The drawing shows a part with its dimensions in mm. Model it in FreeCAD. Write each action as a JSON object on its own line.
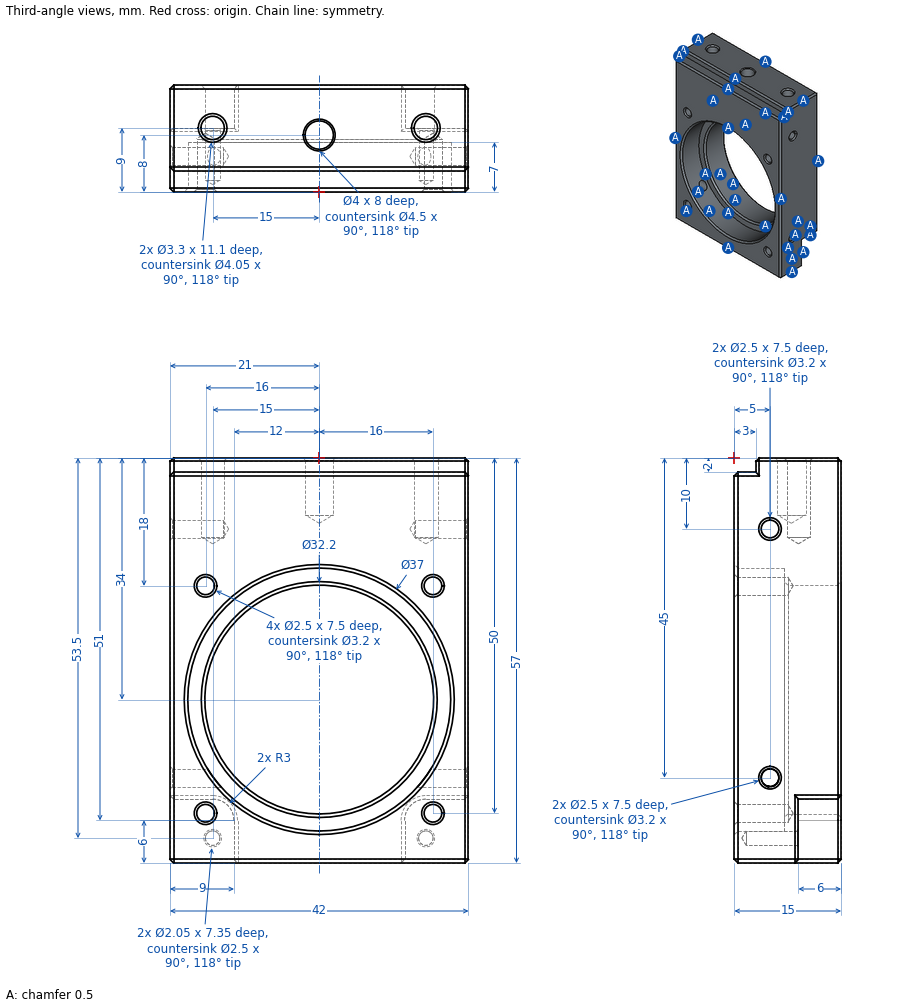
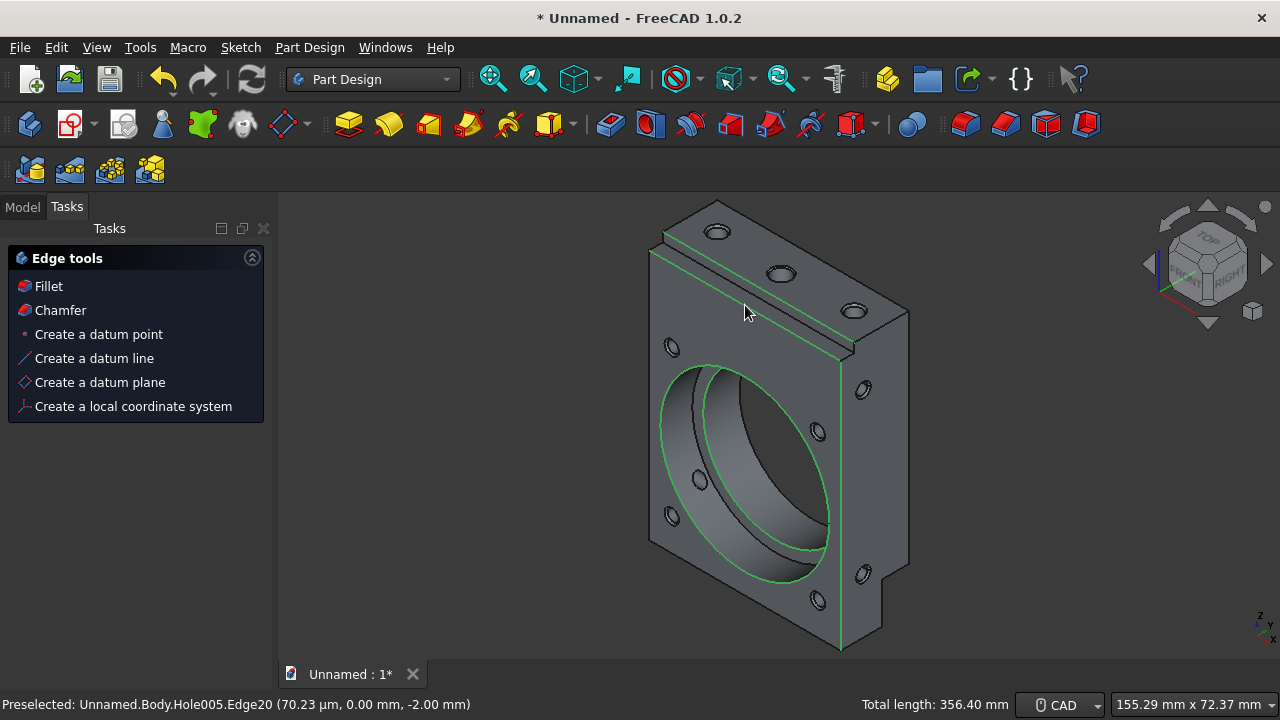
{"action": "left_click", "coordinate": [847, 356], "text": "ctrl"}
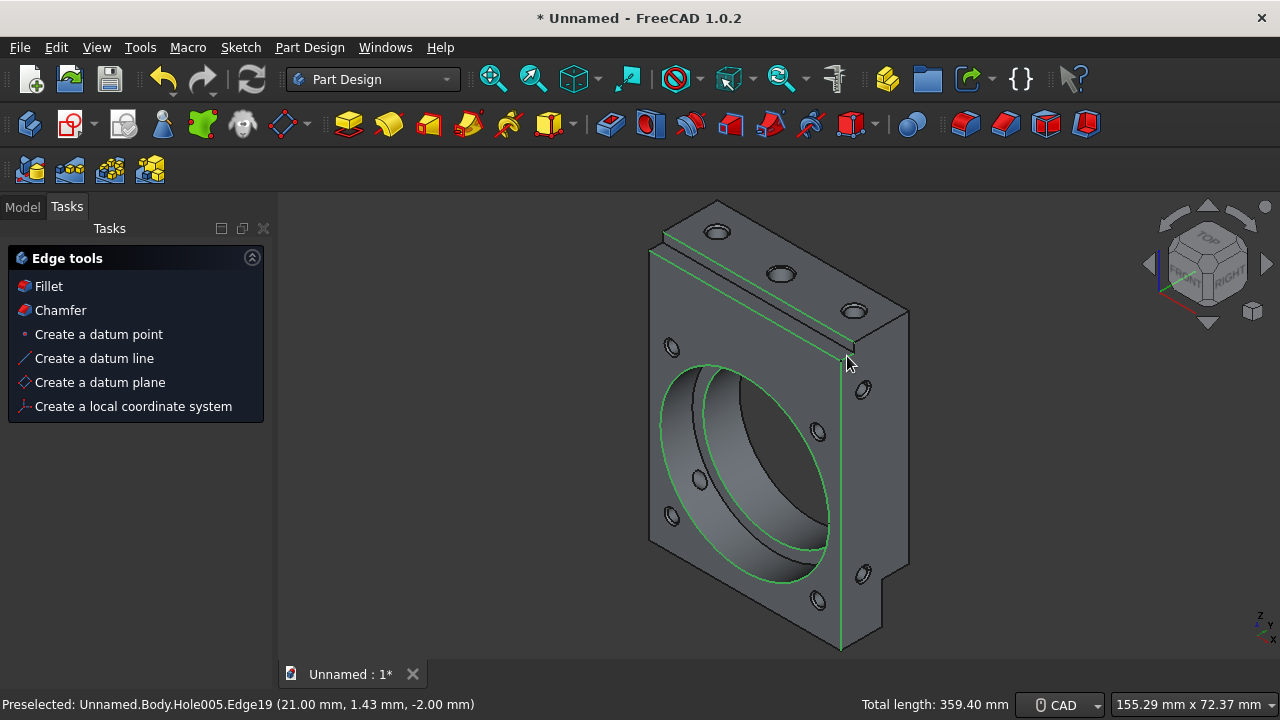
{"action": "left_click", "coordinate": [854, 348], "text": "ctrl"}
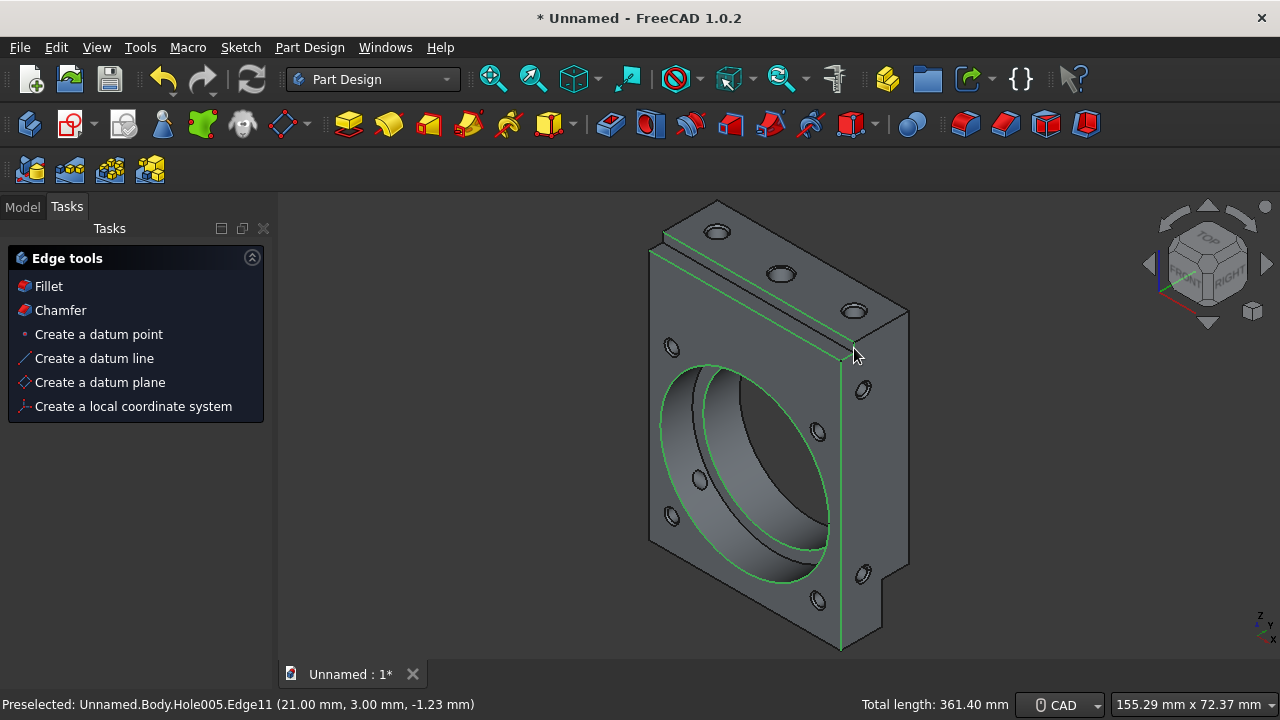
{"action": "left_click", "coordinate": [882, 326], "text": "ctrl"}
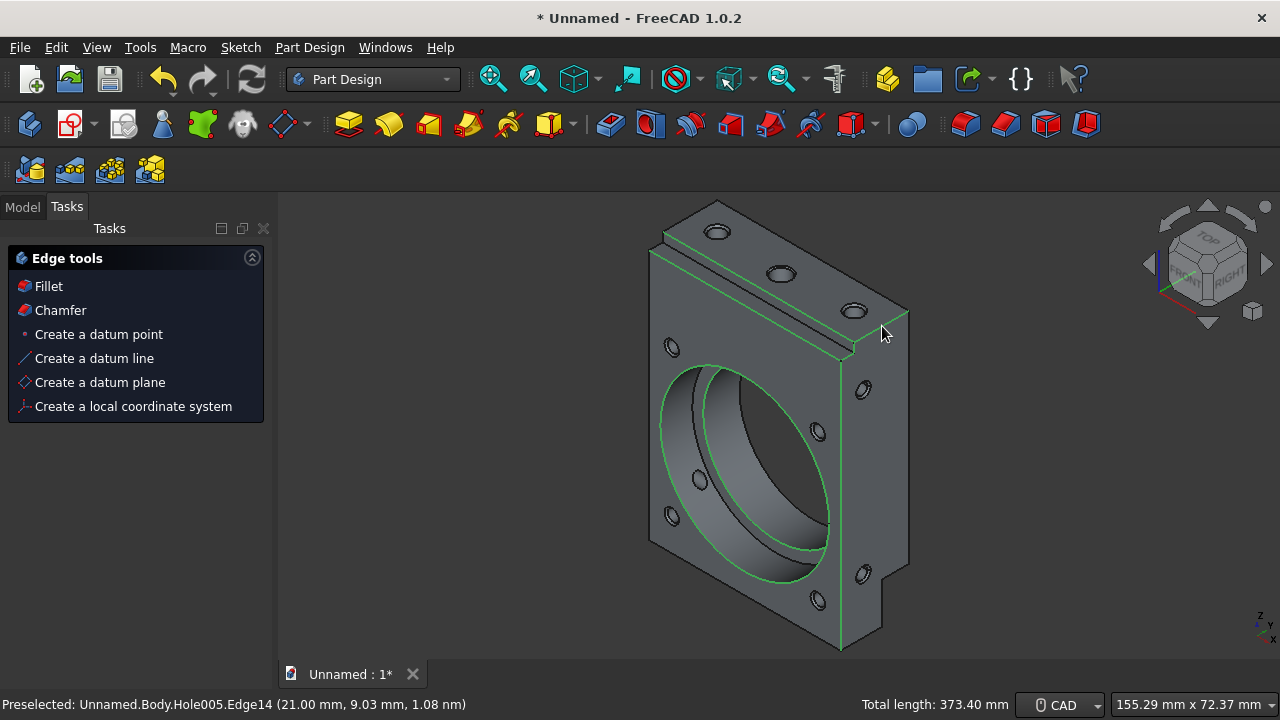
{"action": "key", "text": "2"}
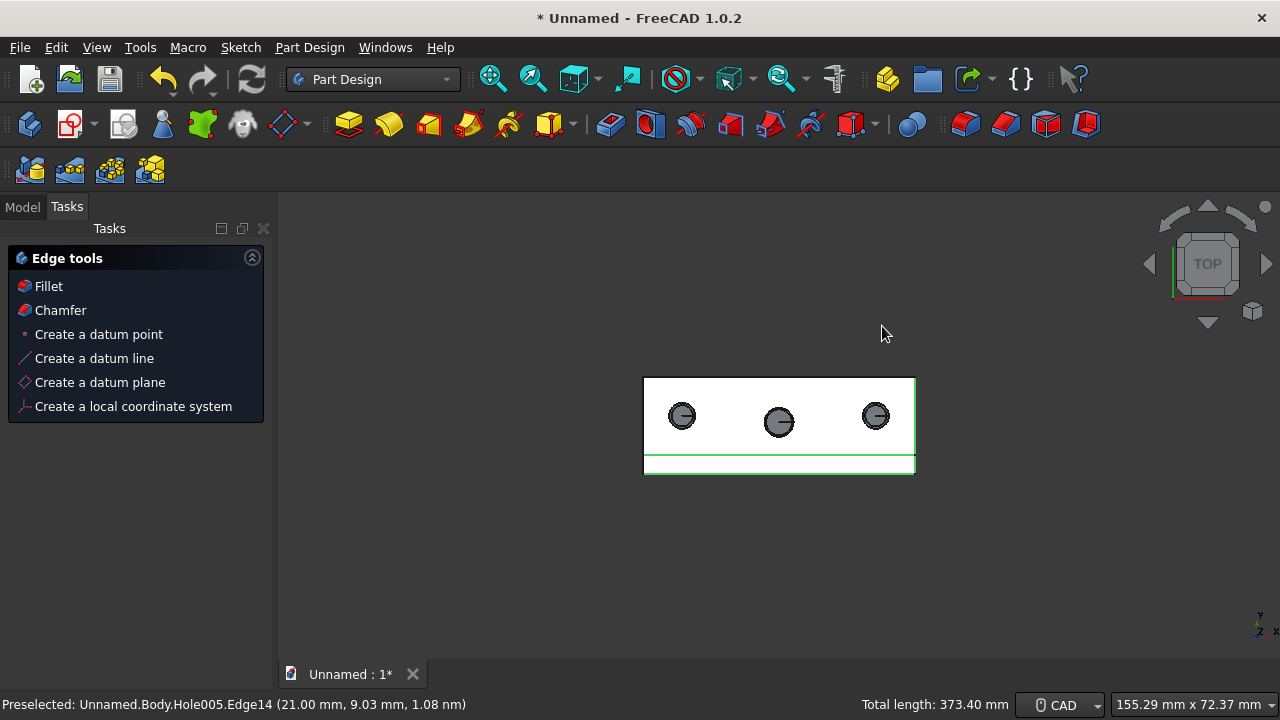
{"action": "key", "text": "v f"}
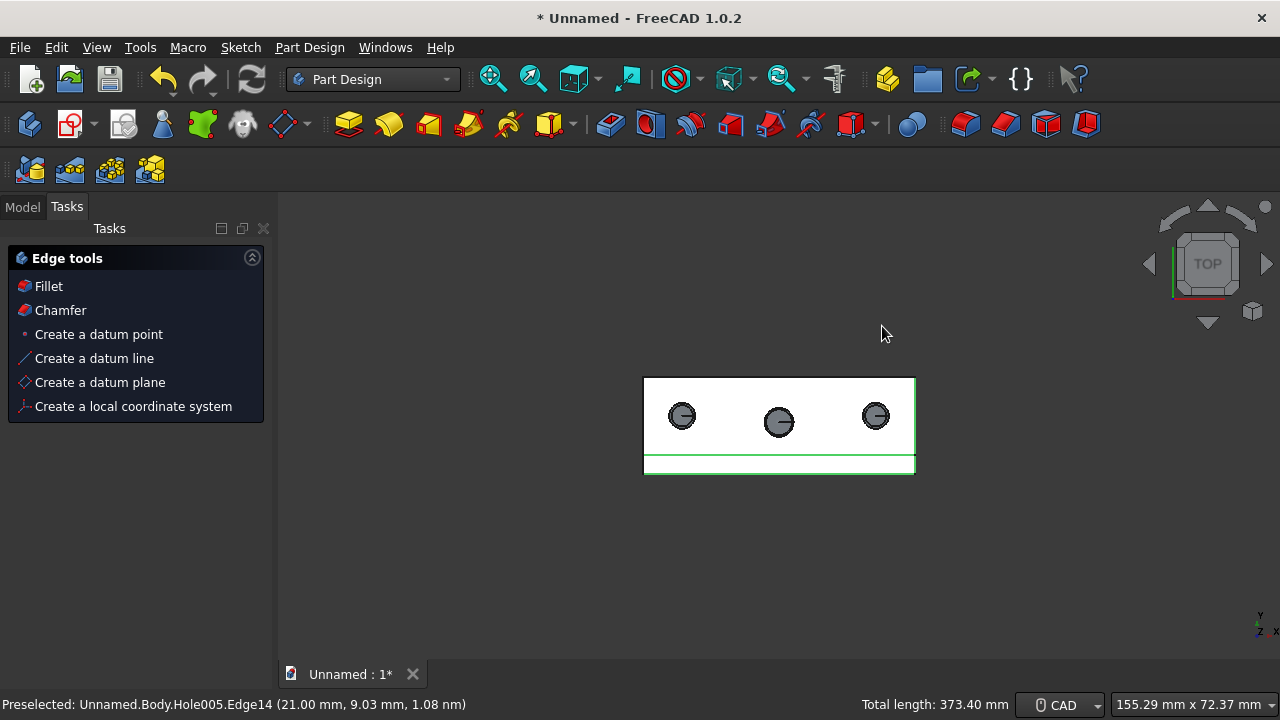
{"action": "left_click", "coordinate": [643, 463], "text": "ctrl"}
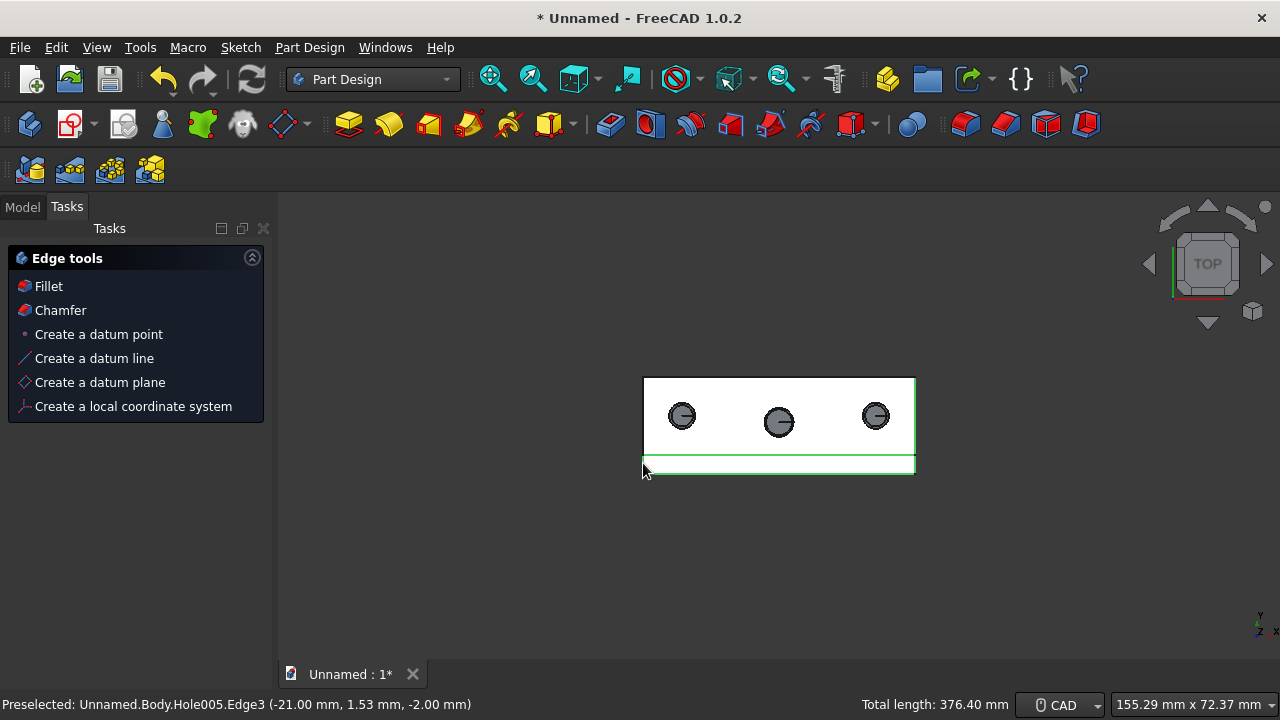
{"action": "left_click", "coordinate": [643, 415], "text": "ctrl"}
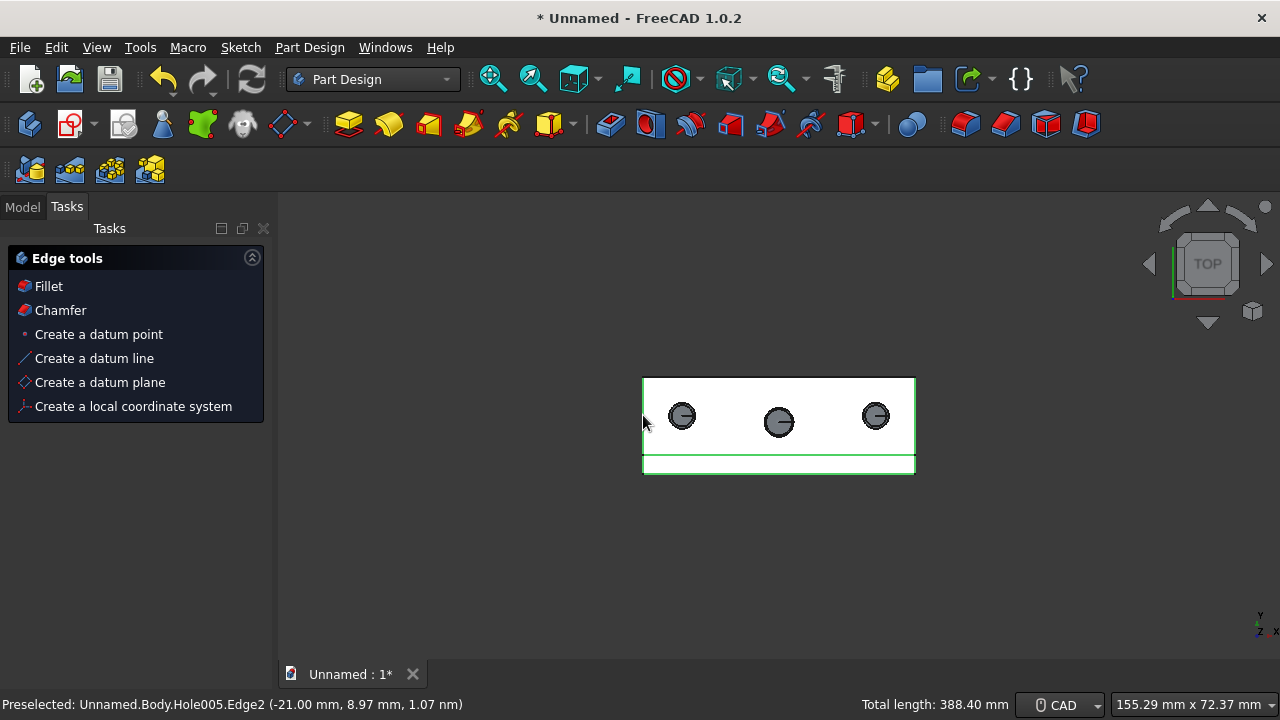
{"action": "key", "text": "0"}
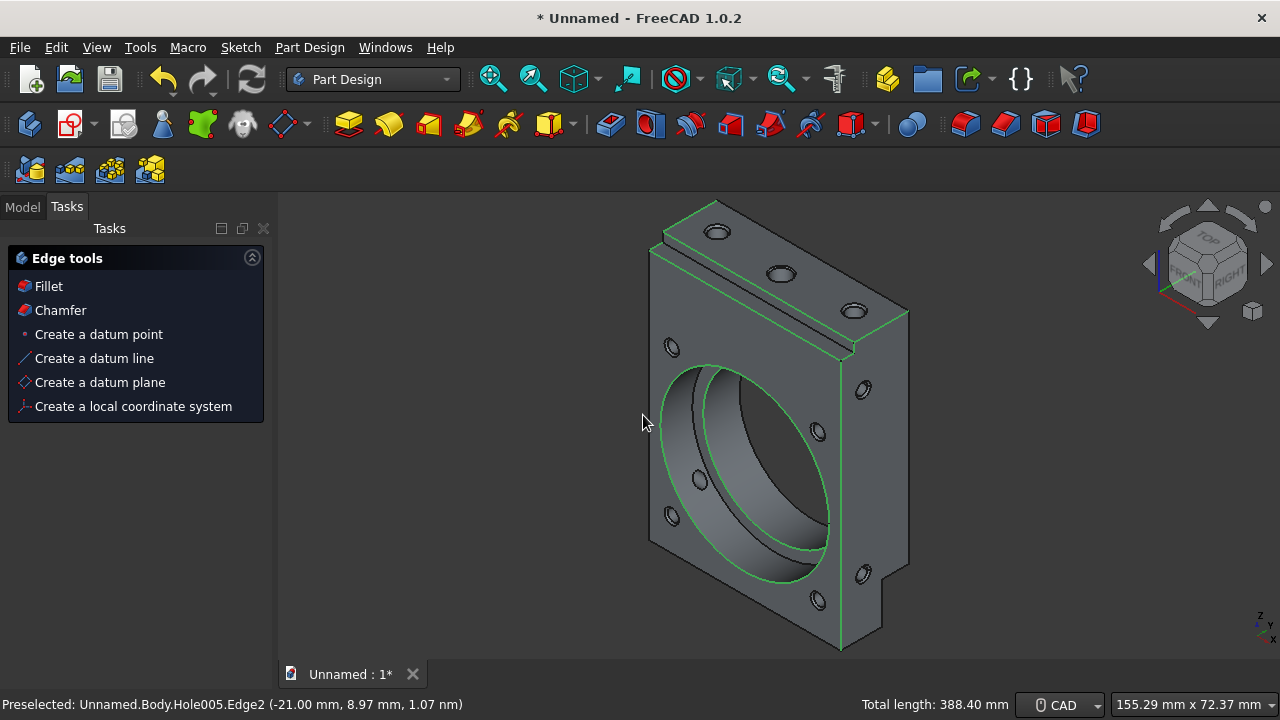
{"action": "key", "text": "1"}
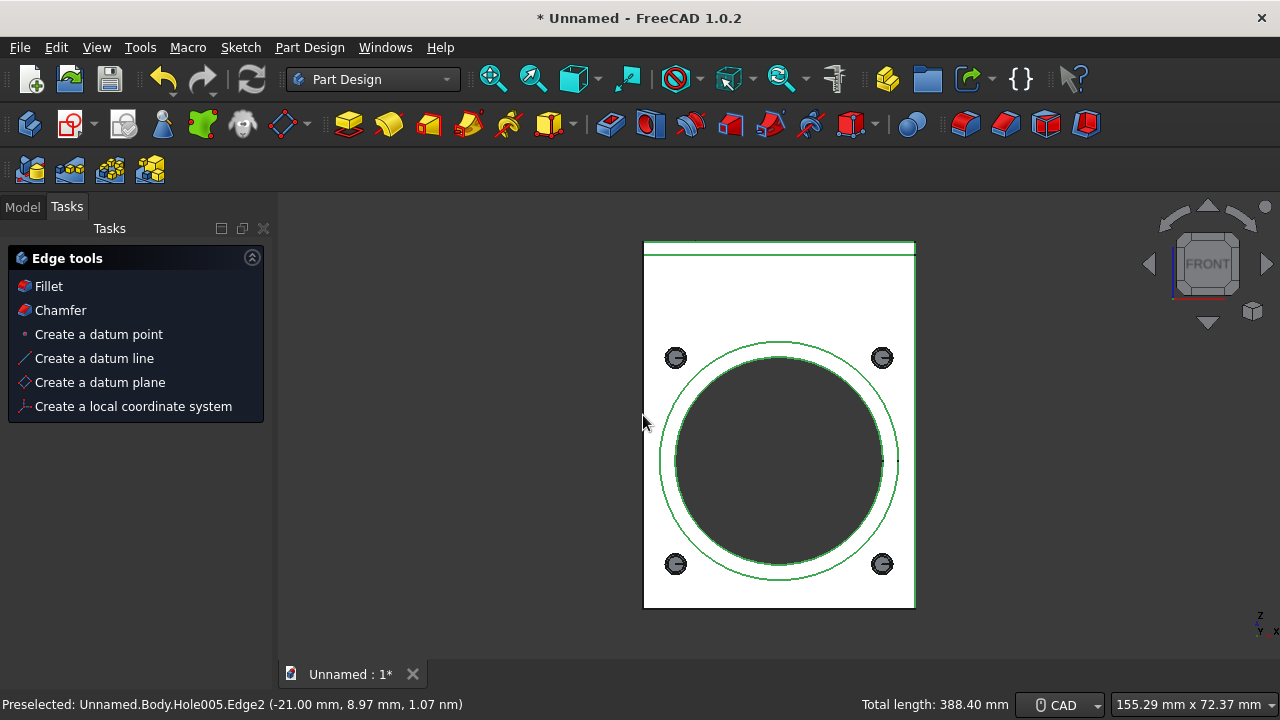
{"action": "left_click", "coordinate": [643, 247], "text": "ctrl"}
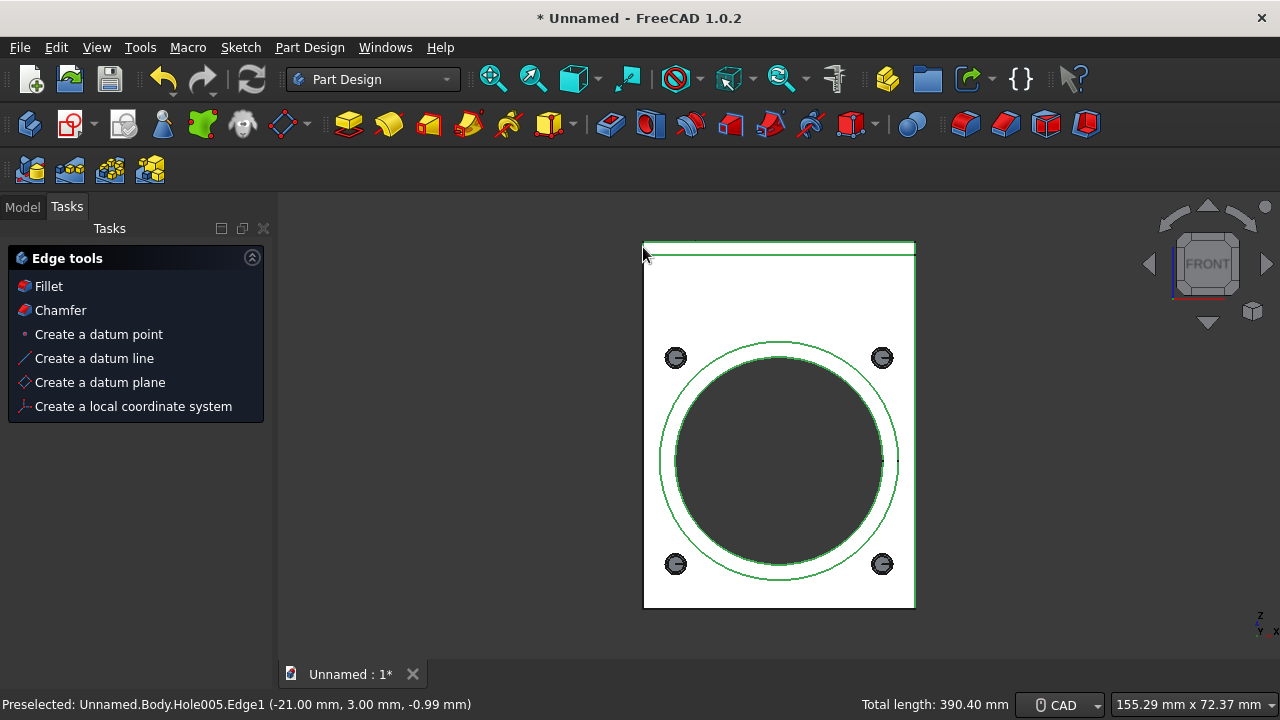
{"action": "key", "text": "3"}